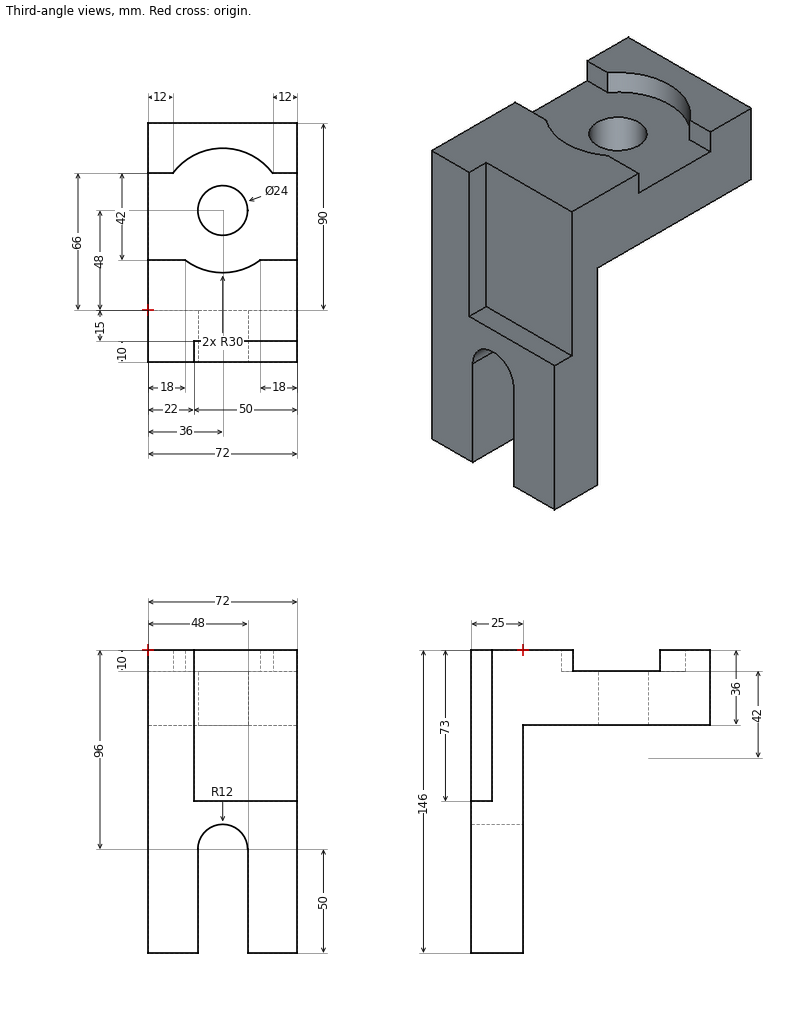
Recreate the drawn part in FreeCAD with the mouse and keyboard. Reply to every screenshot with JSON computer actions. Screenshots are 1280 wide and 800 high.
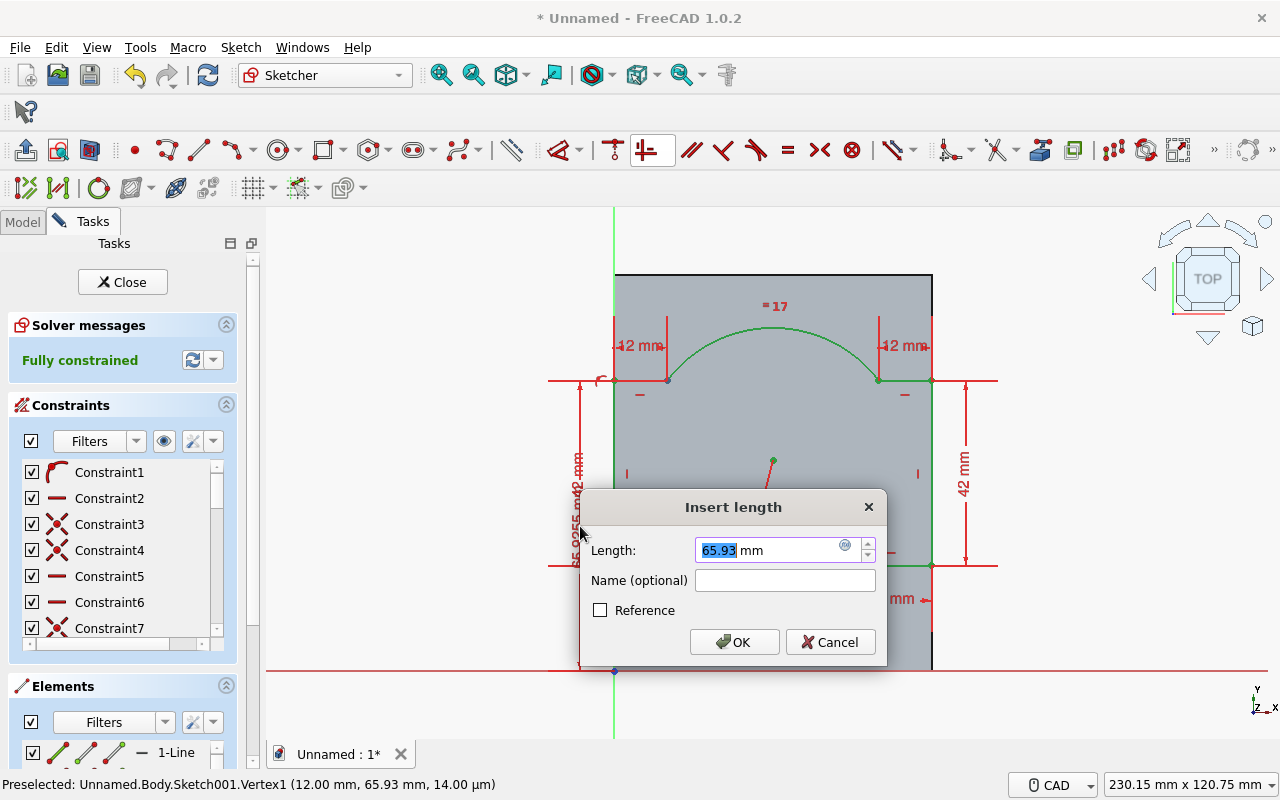
{"action": "type", "text": "66"}
{"action": "key", "text": "Return"}
{"action": "key", "text": "Escape"}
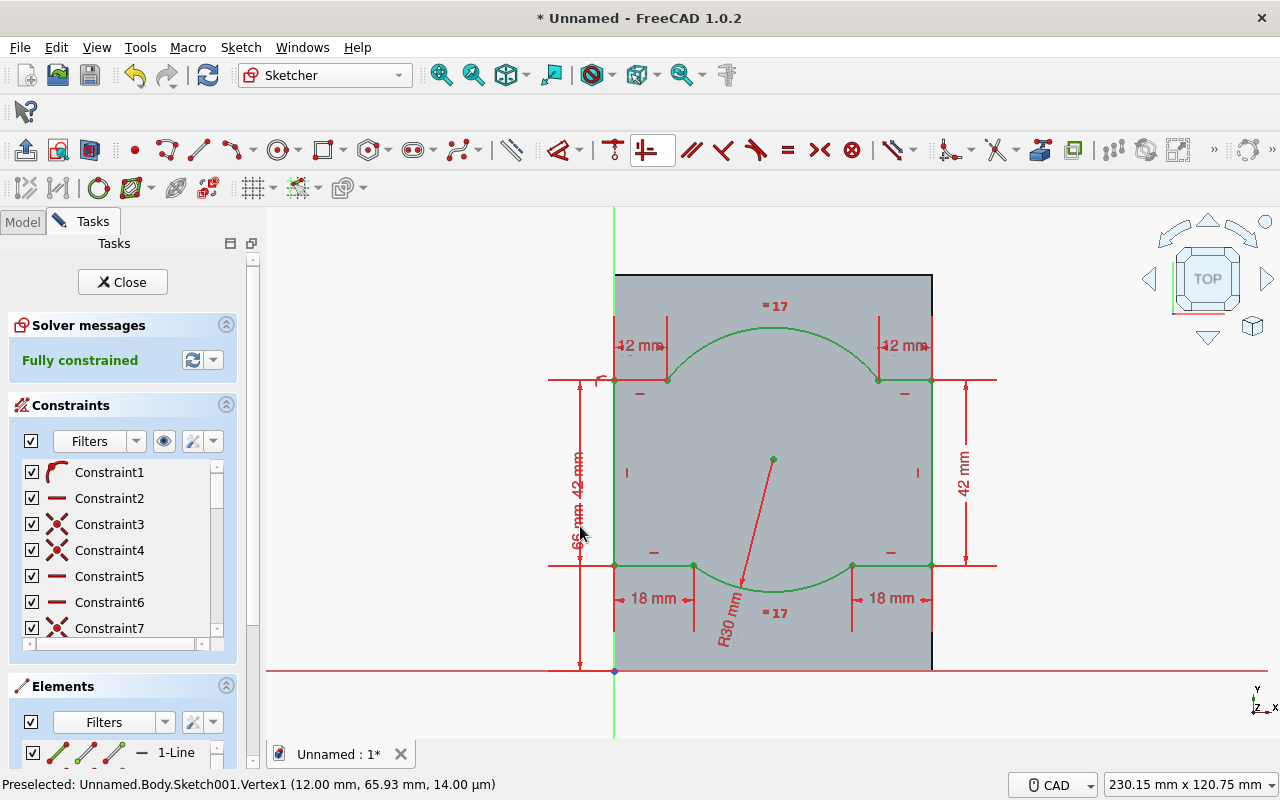
{"action": "left_click", "coordinate": [123, 282]}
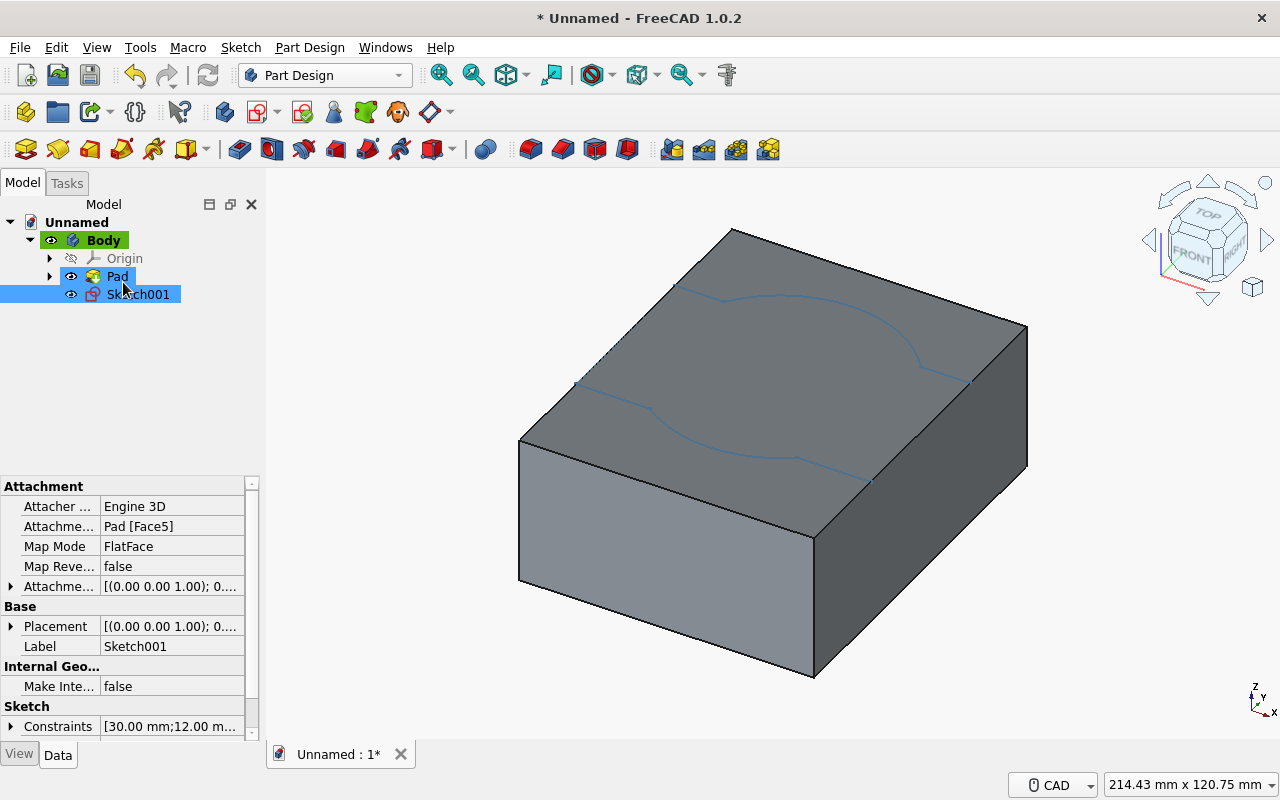
{"action": "left_click", "coordinate": [240, 150]}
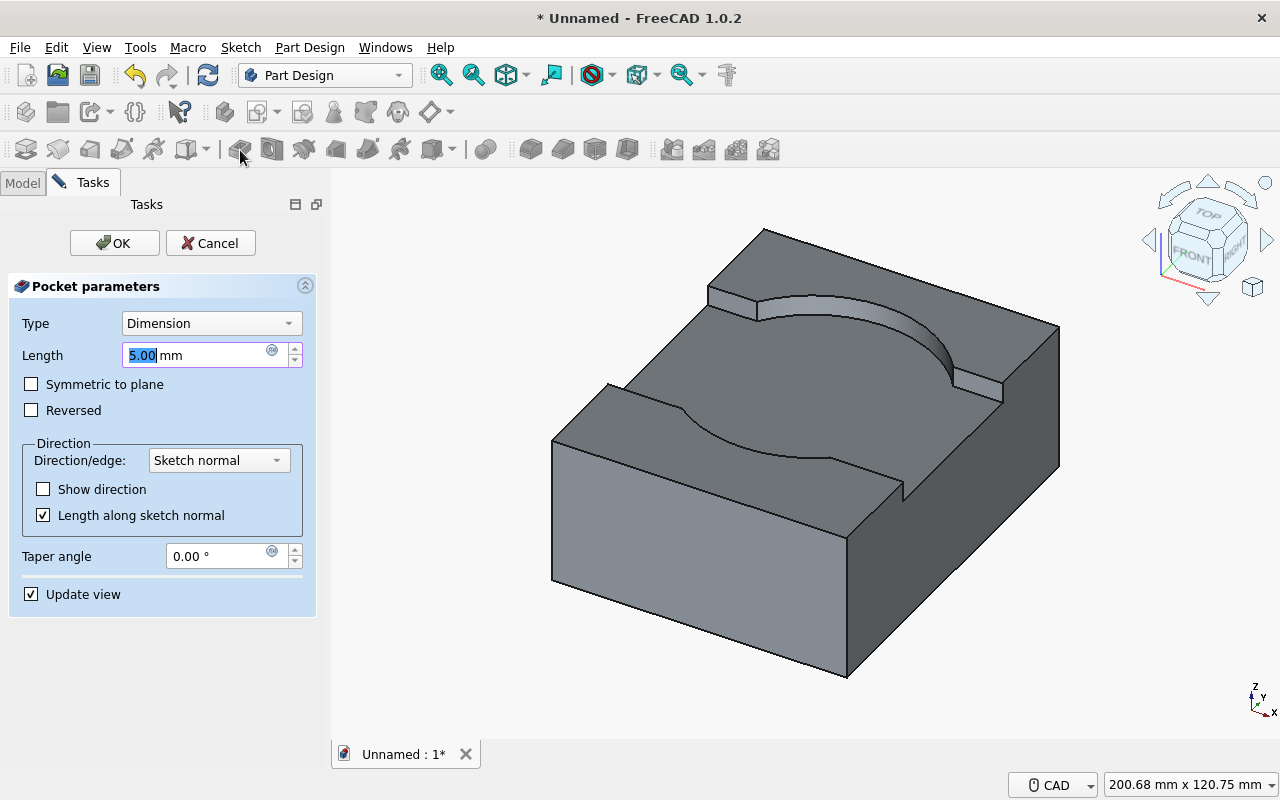
{"action": "type", "text": "10"}
{"action": "key", "text": "Tab"}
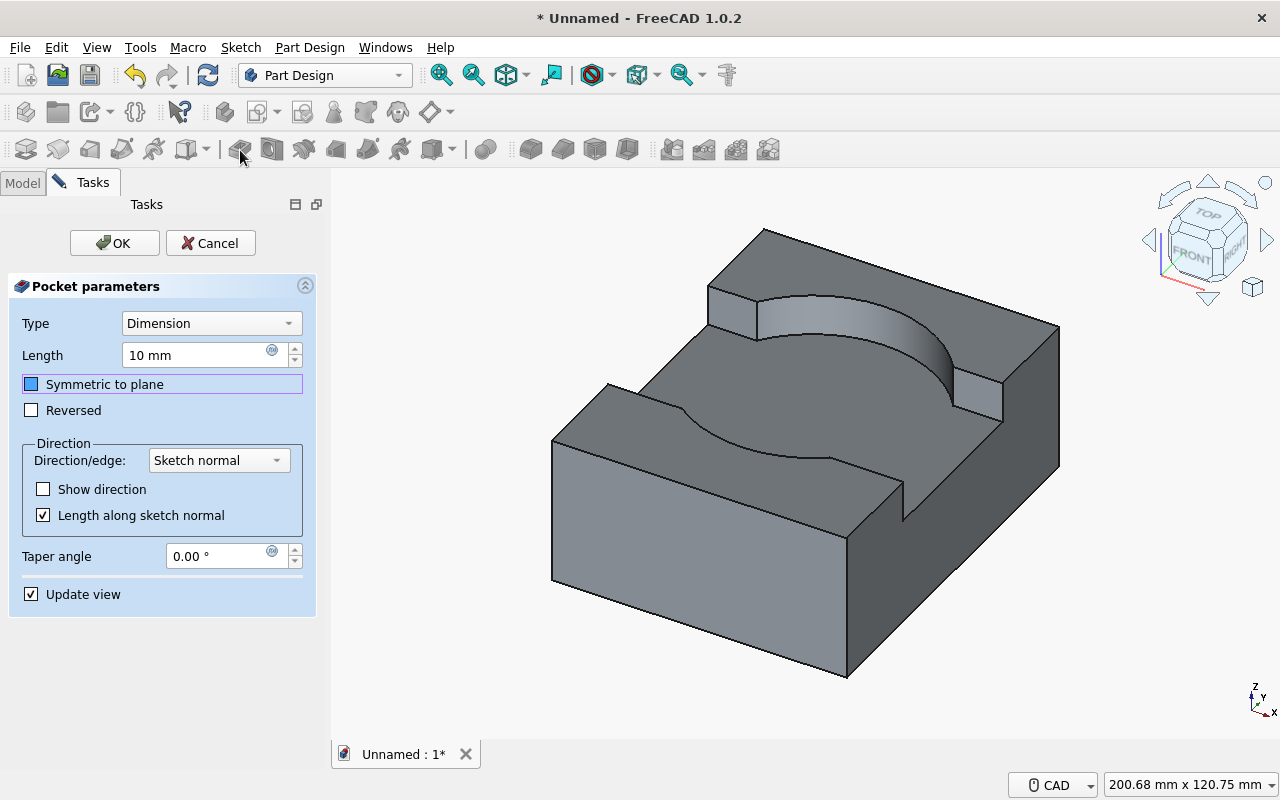
{"action": "left_click", "coordinate": [115, 243]}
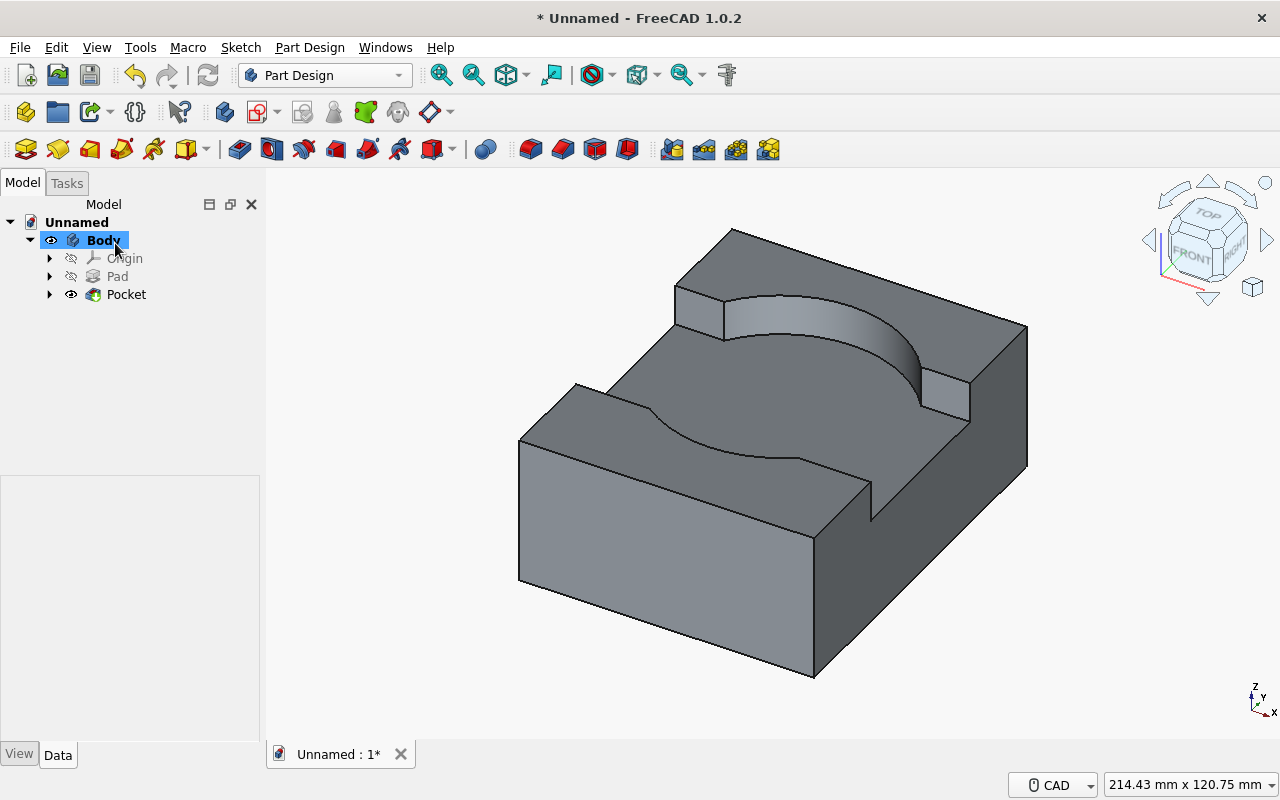
{"action": "left_click", "coordinate": [780, 414]}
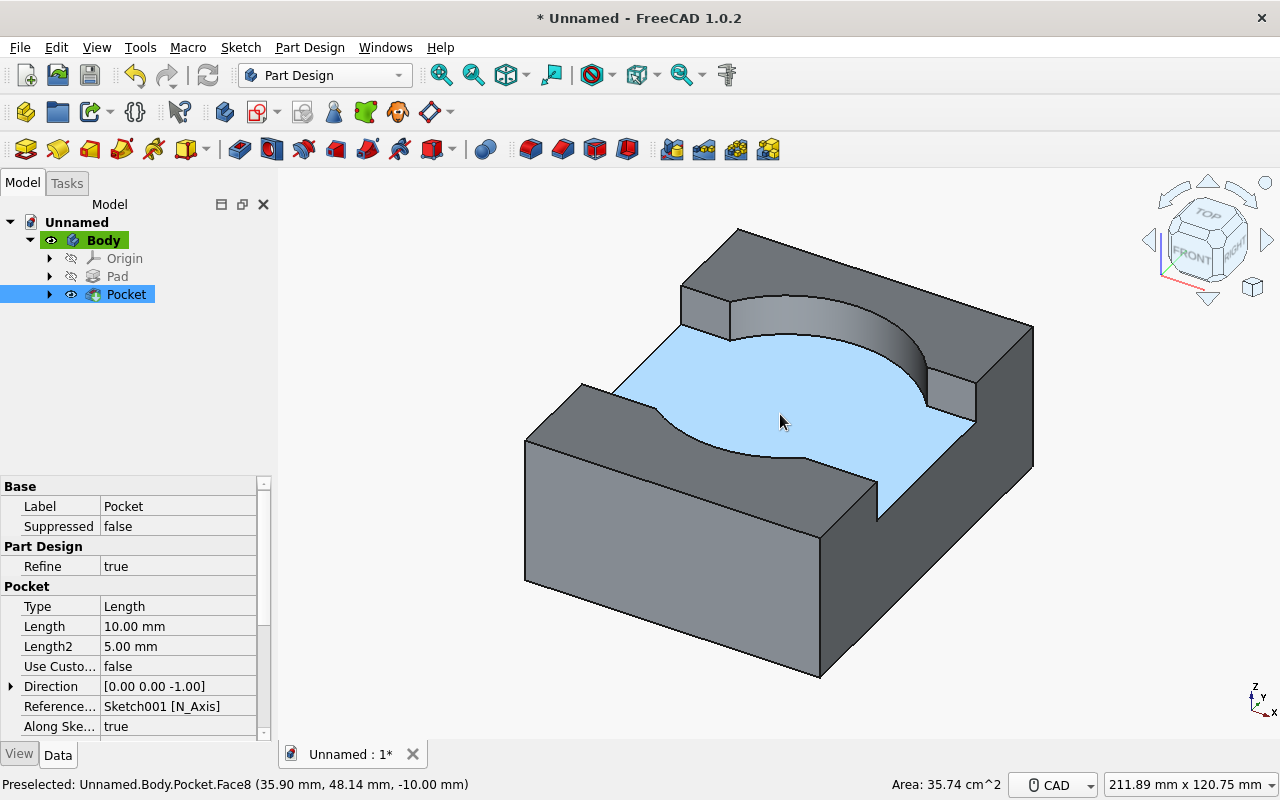
{"action": "left_click", "coordinate": [258, 112]}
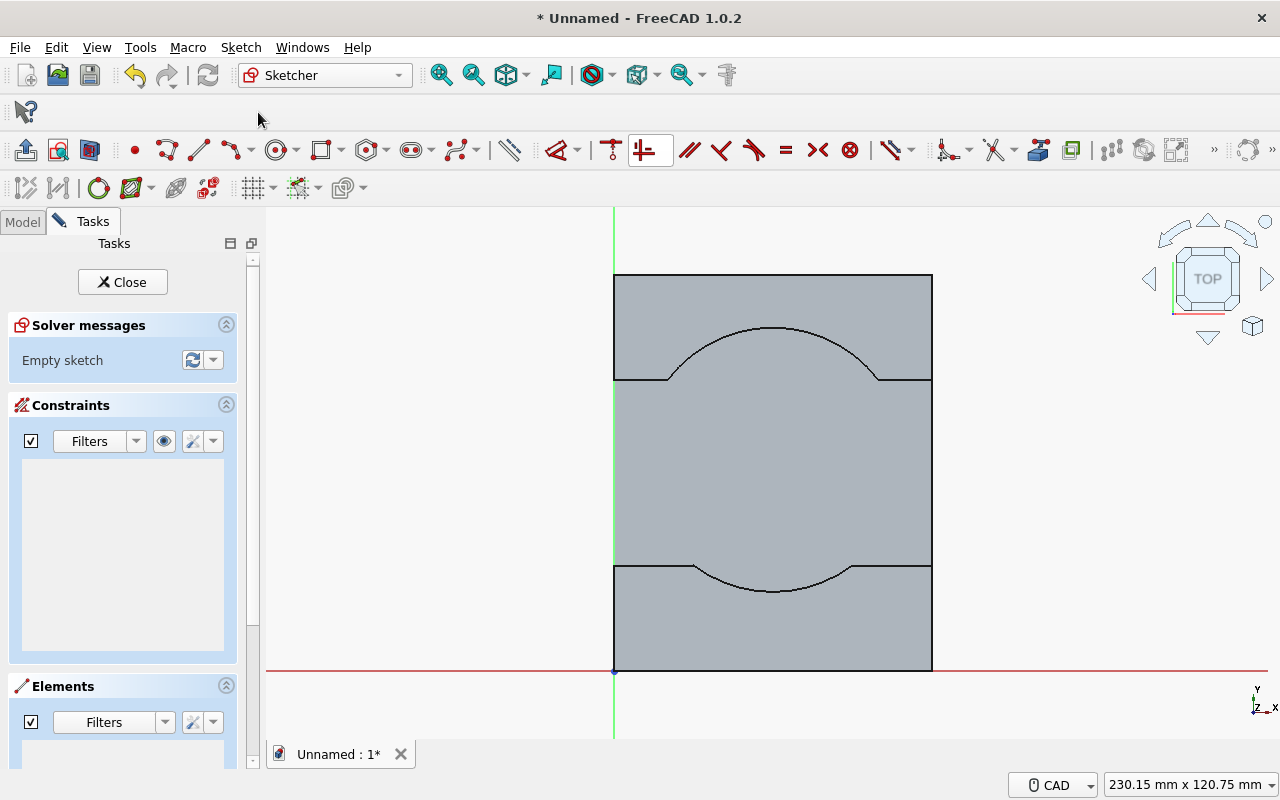
{"action": "left_click", "coordinate": [90, 150]}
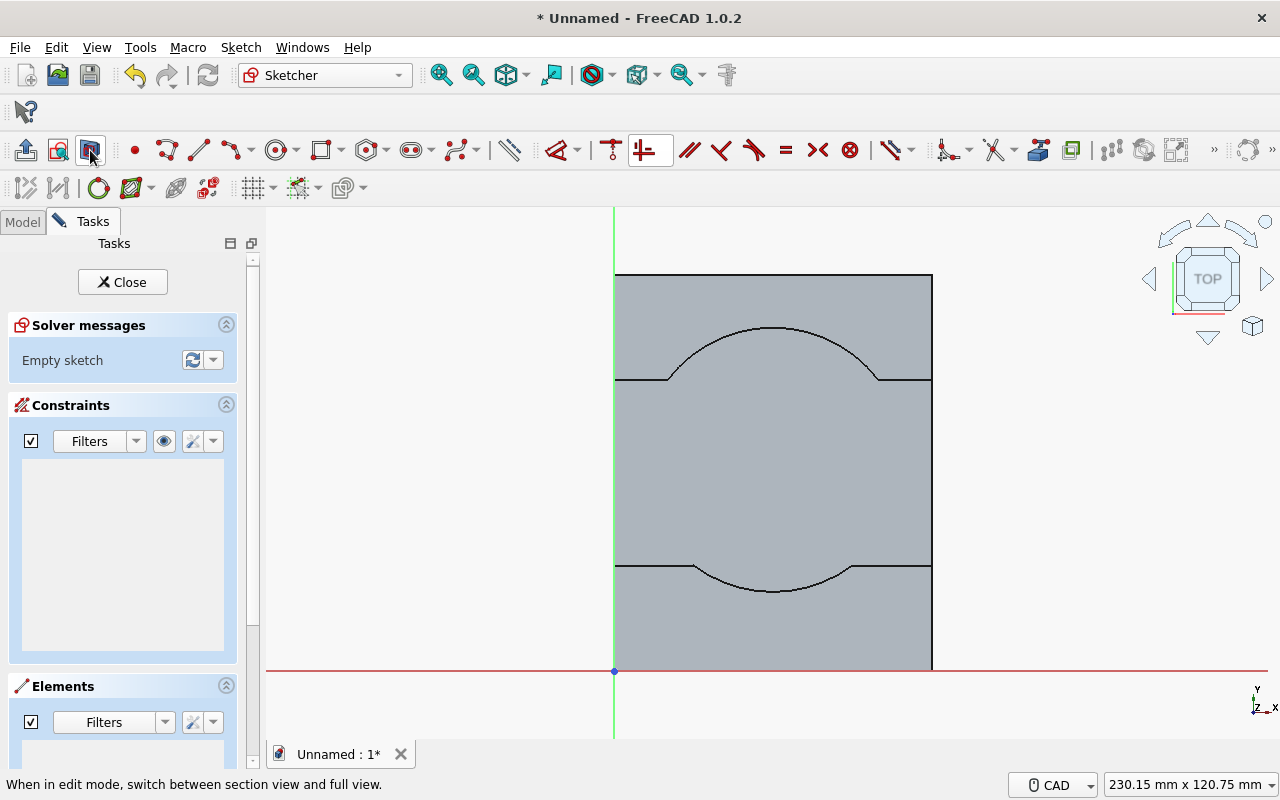
{"action": "scroll", "coordinate": [803, 454], "scroll_direction": "up", "scroll_amount": 6}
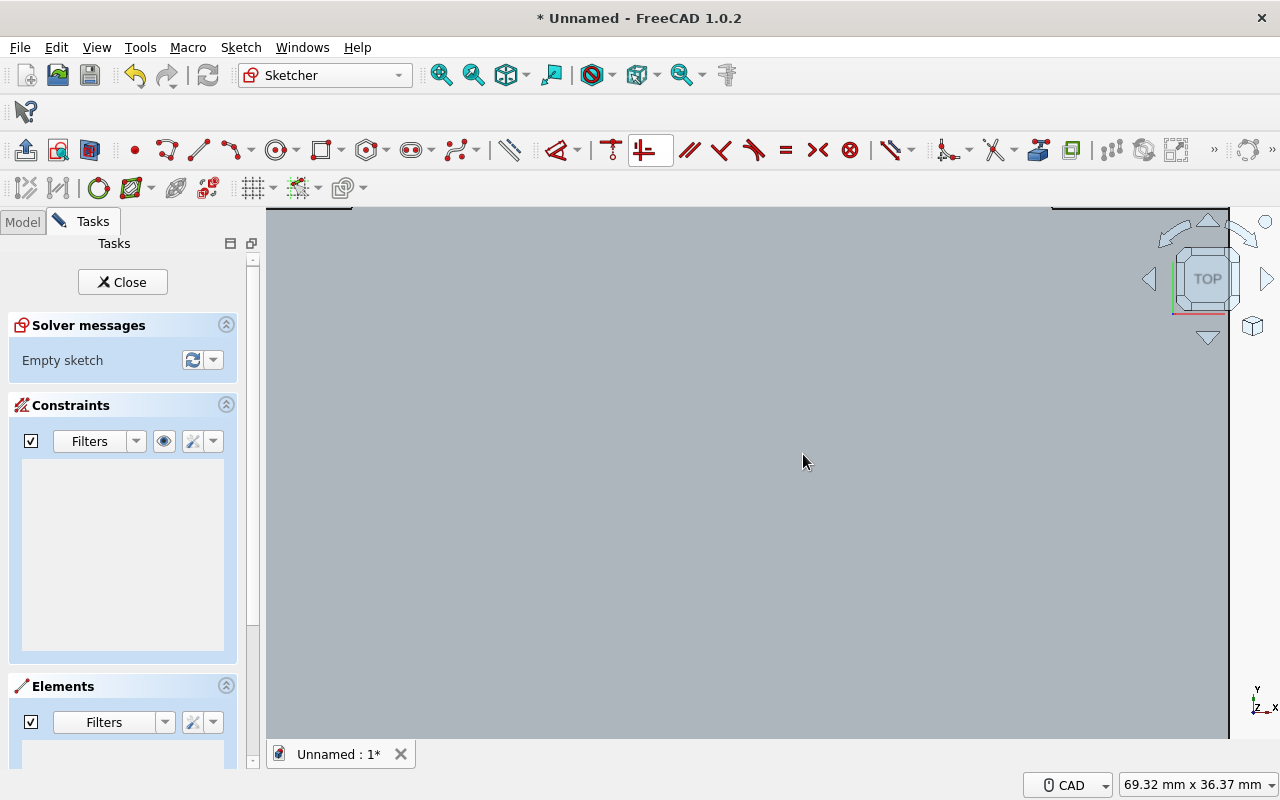
{"action": "left_click", "coordinate": [276, 150]}